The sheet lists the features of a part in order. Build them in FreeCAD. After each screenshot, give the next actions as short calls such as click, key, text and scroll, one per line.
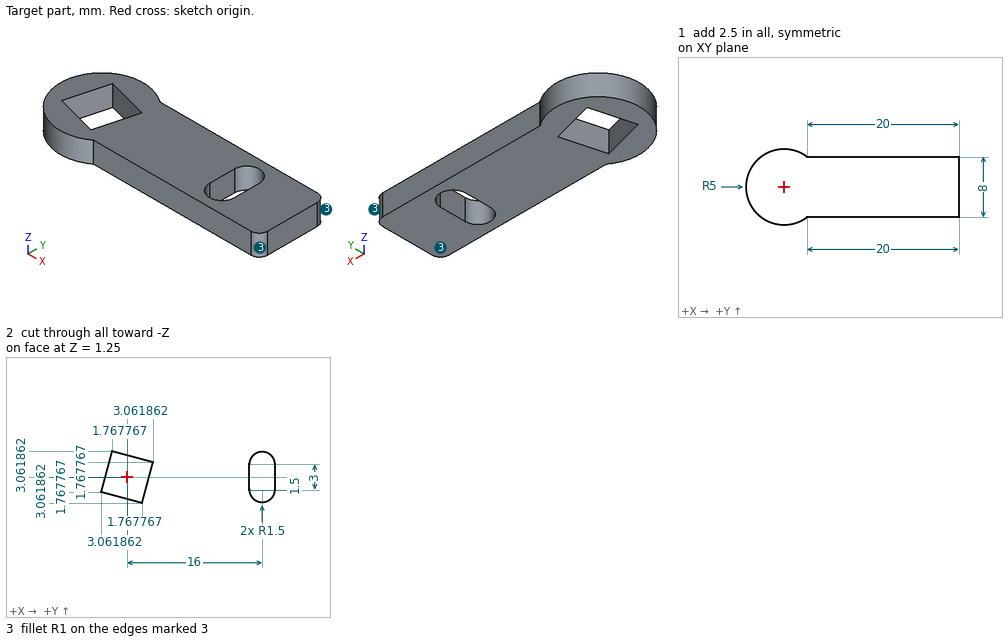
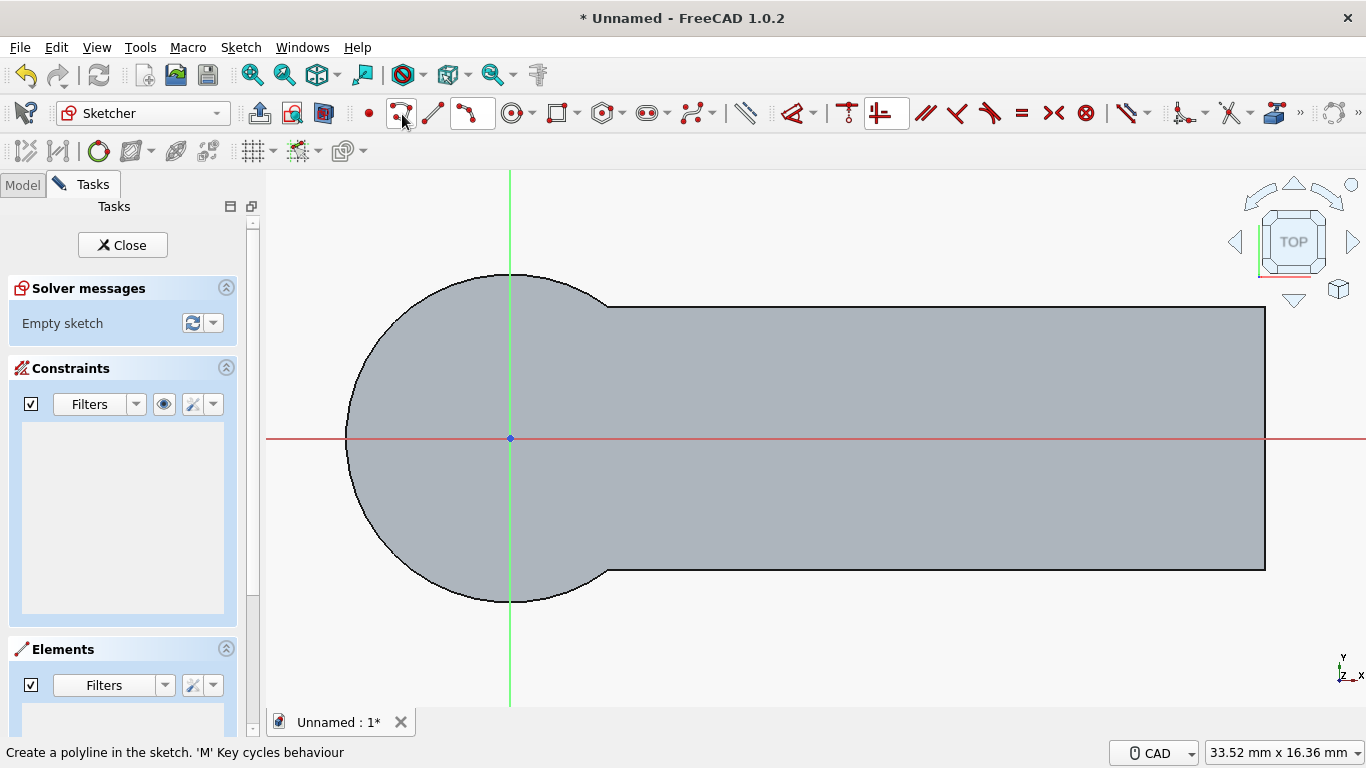
click(568, 539)
click(611, 380)
click(452, 338)
click(410, 497)
click(568, 540)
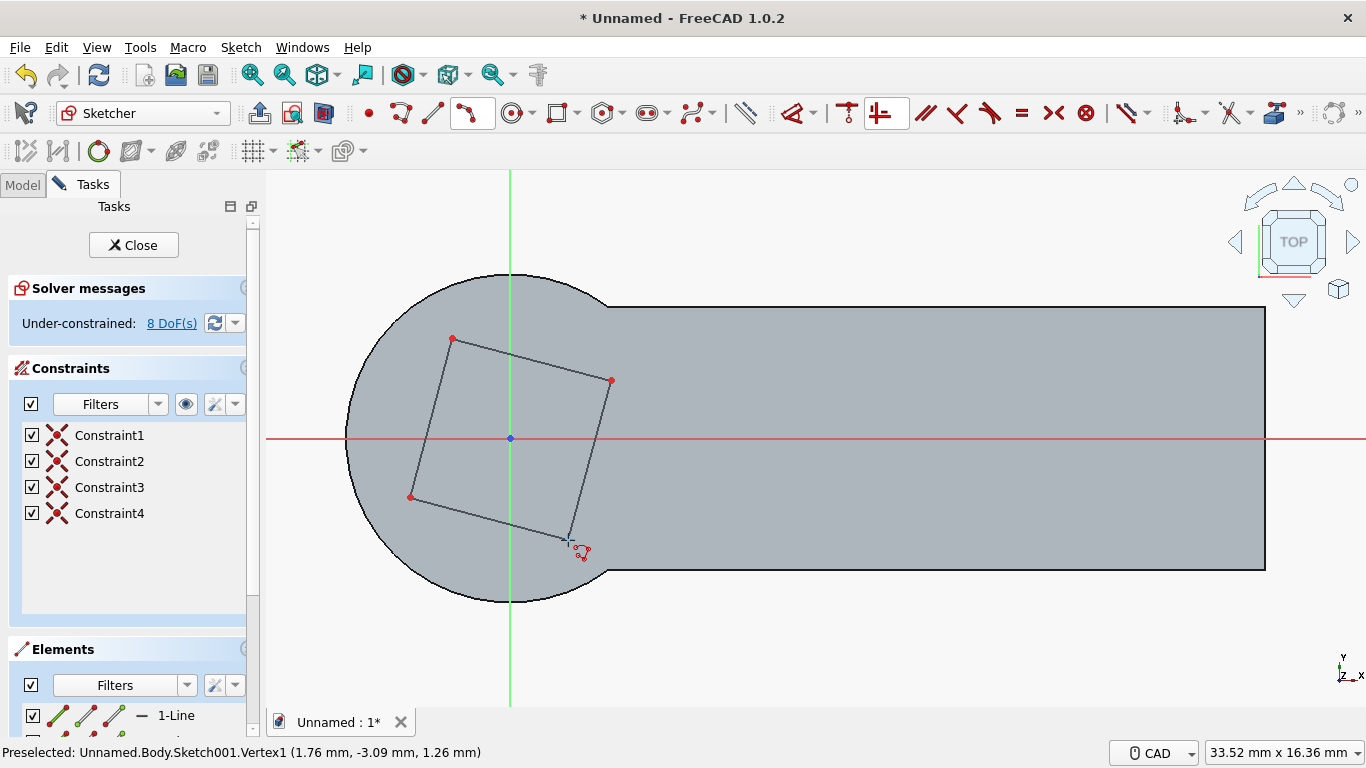
click(648, 114)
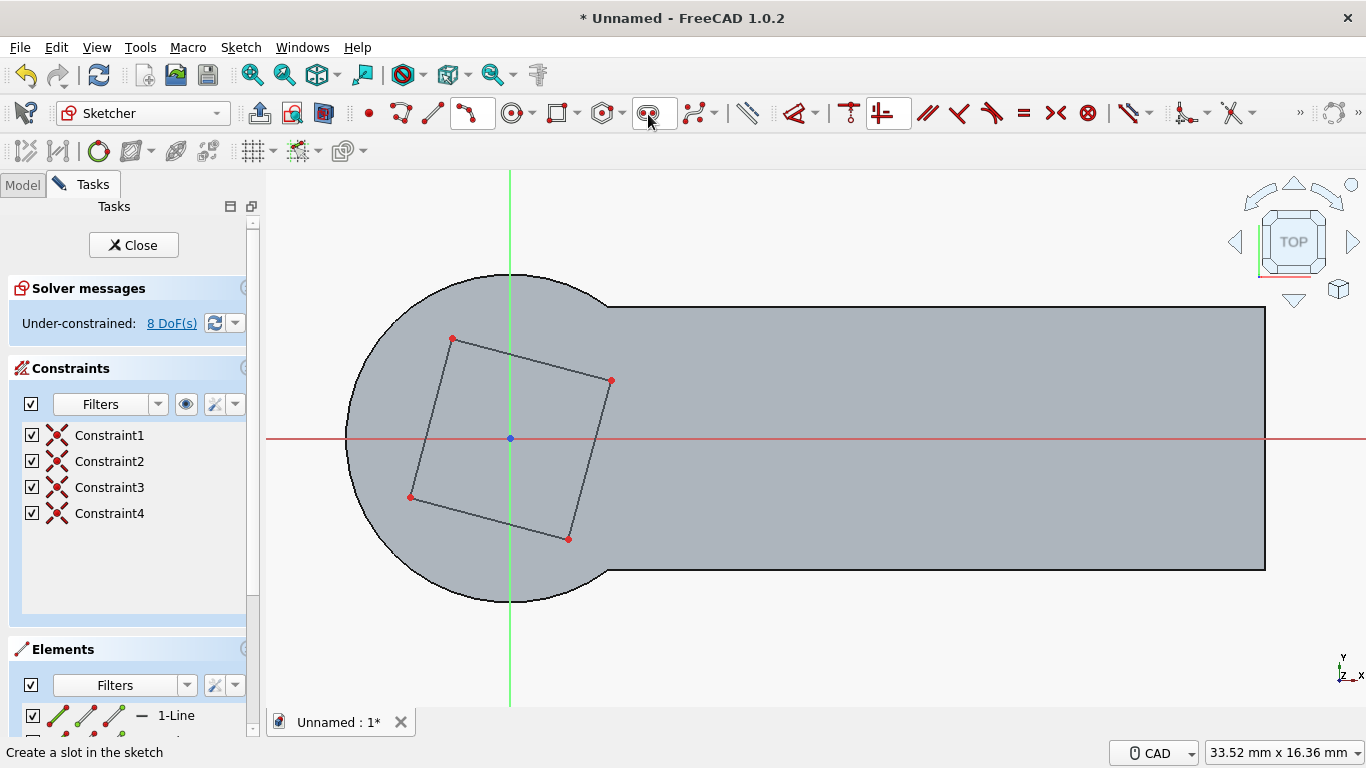
click(1035, 488)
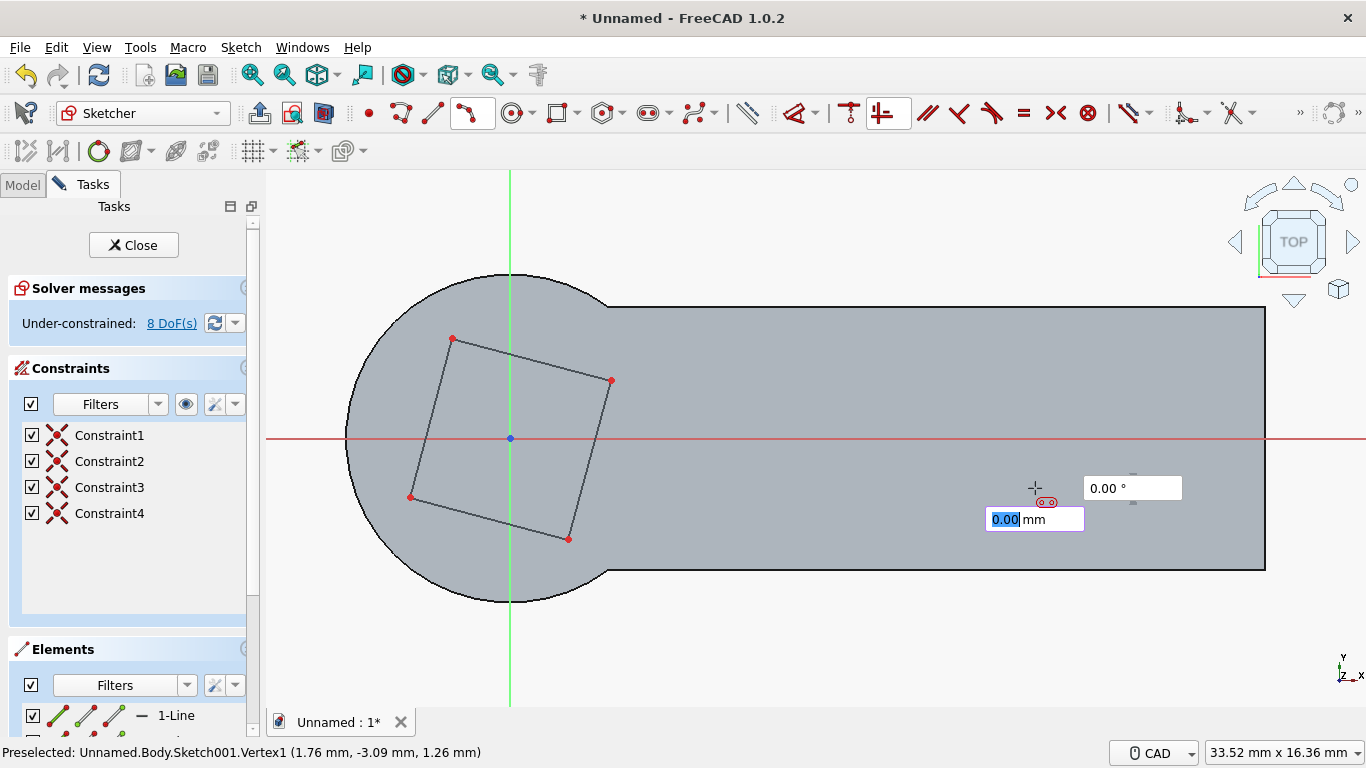
click(1035, 389)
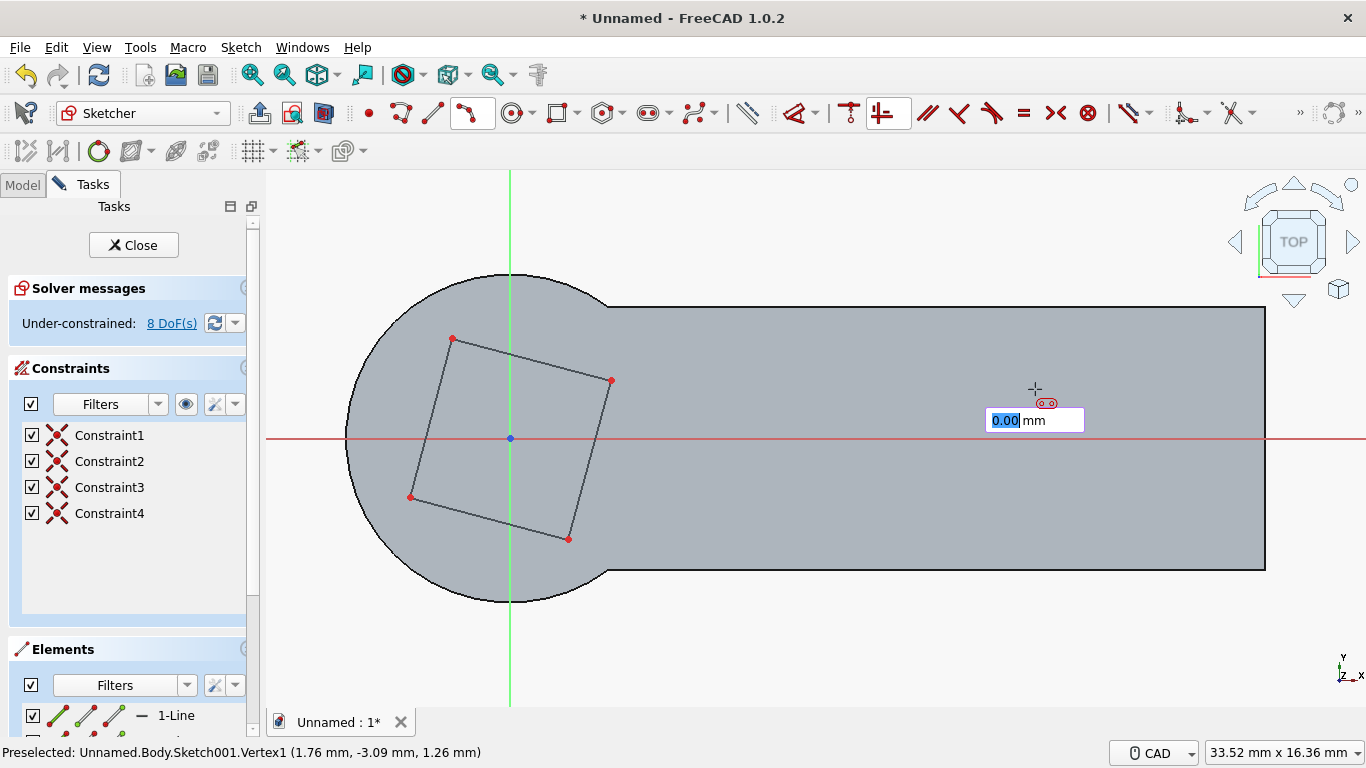
click(986, 424)
key(Escape)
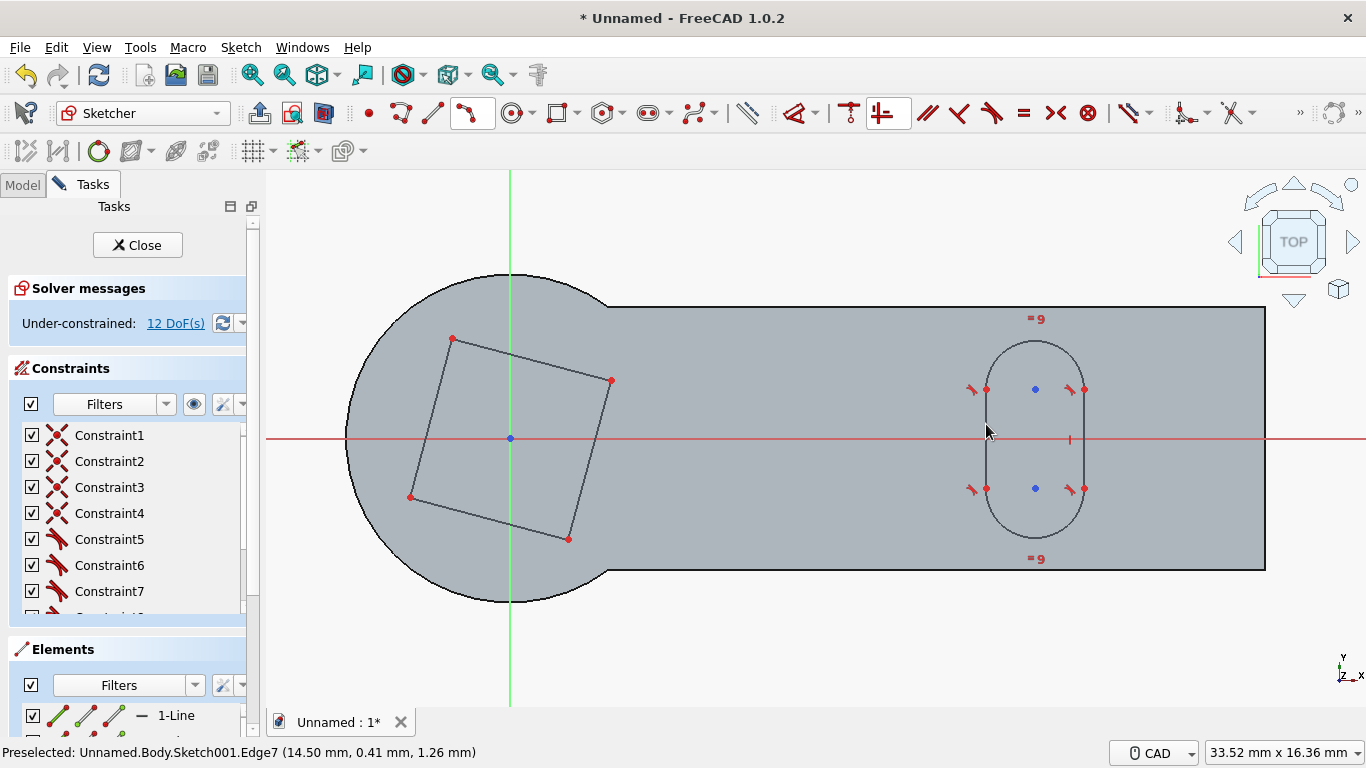
click(794, 114)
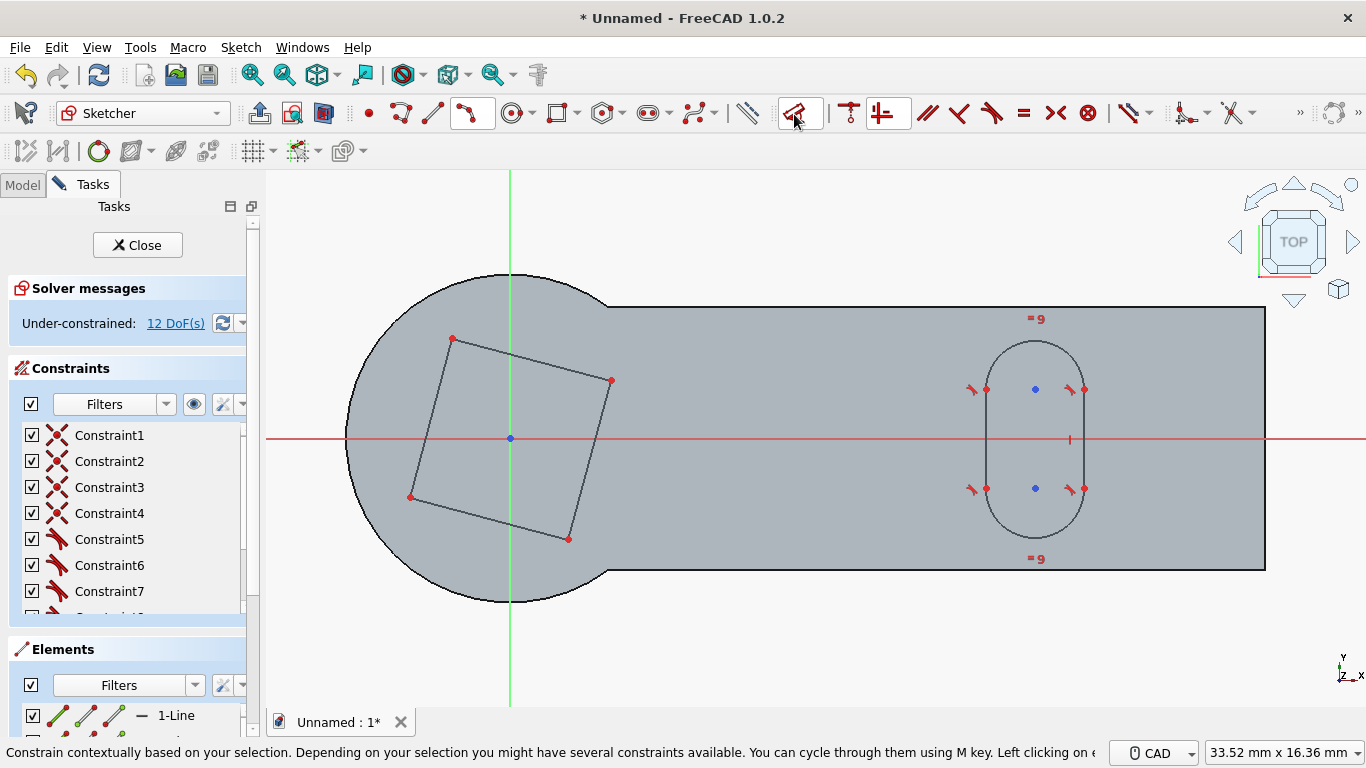
click(1006, 529)
click(987, 555)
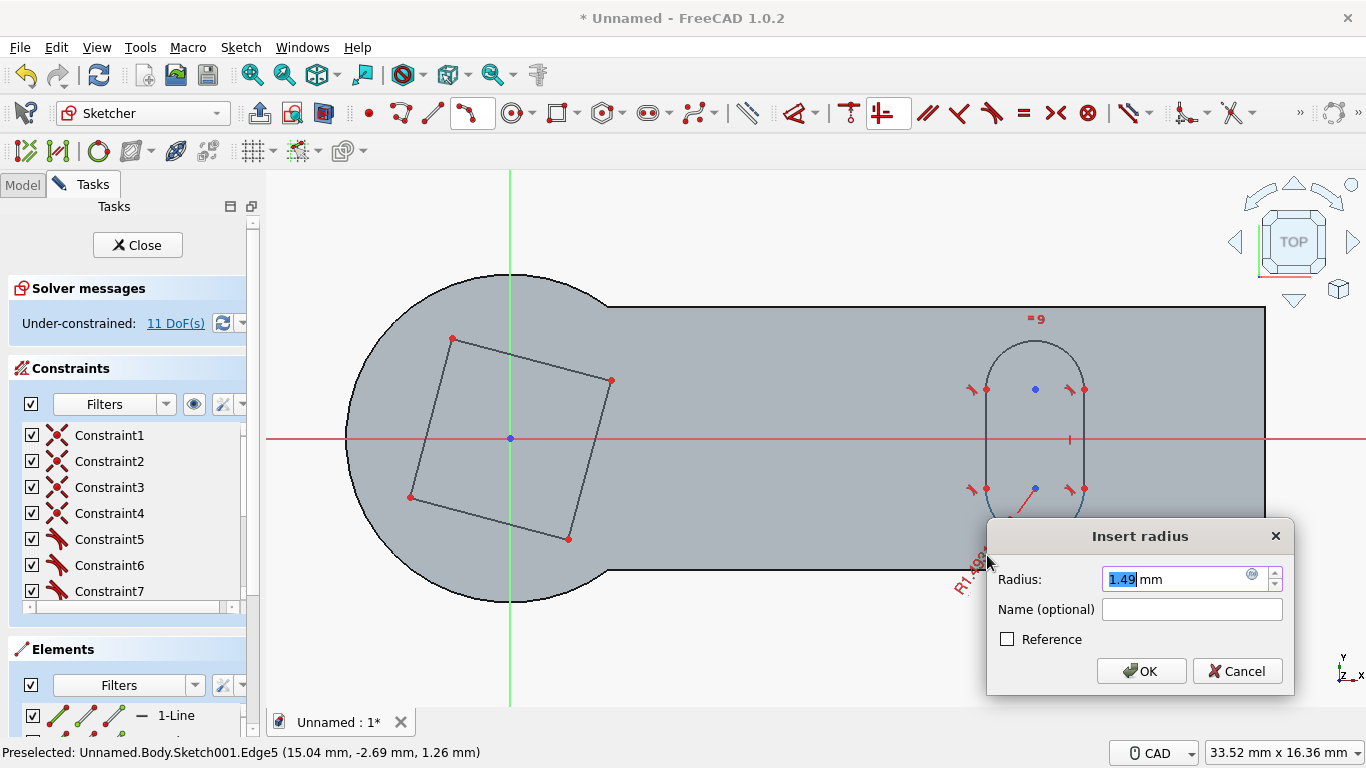
text(1.5)
key(Return)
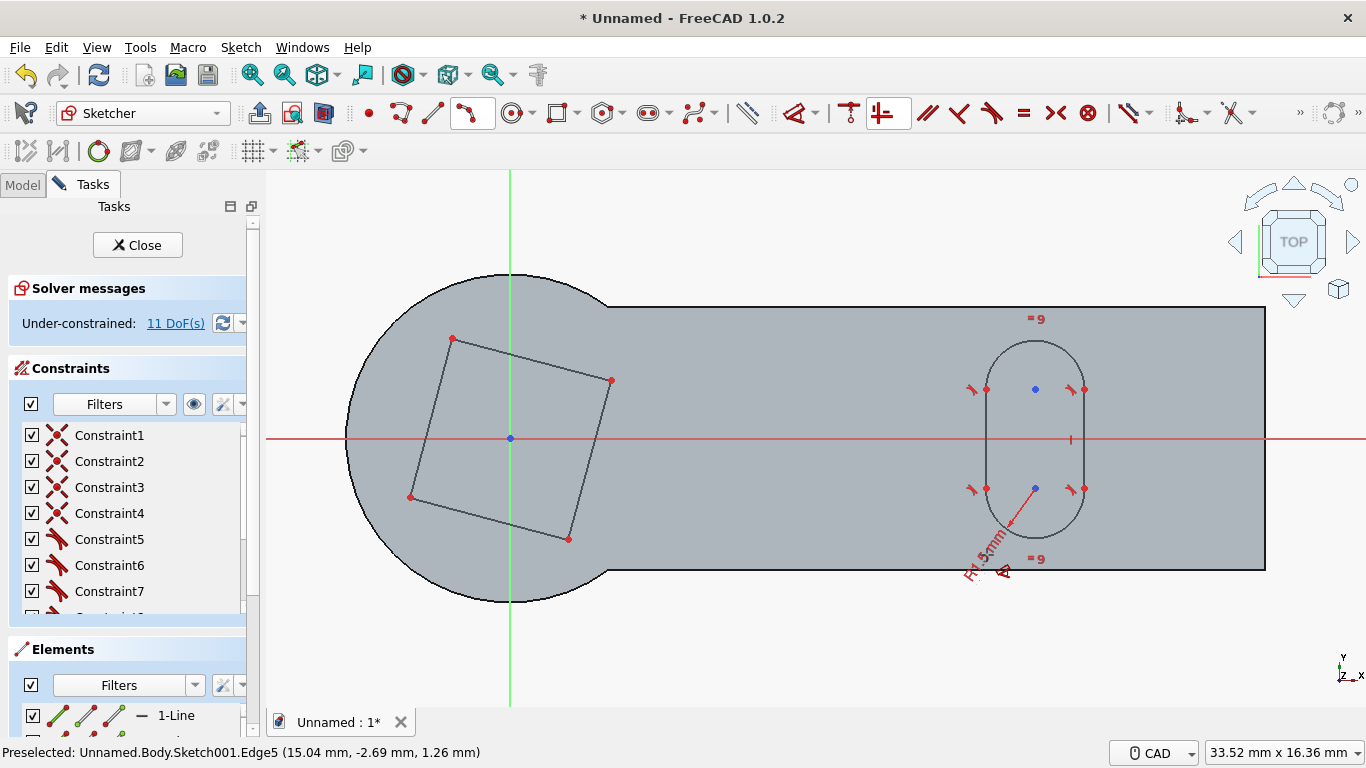
click(986, 459)
click(1020, 417)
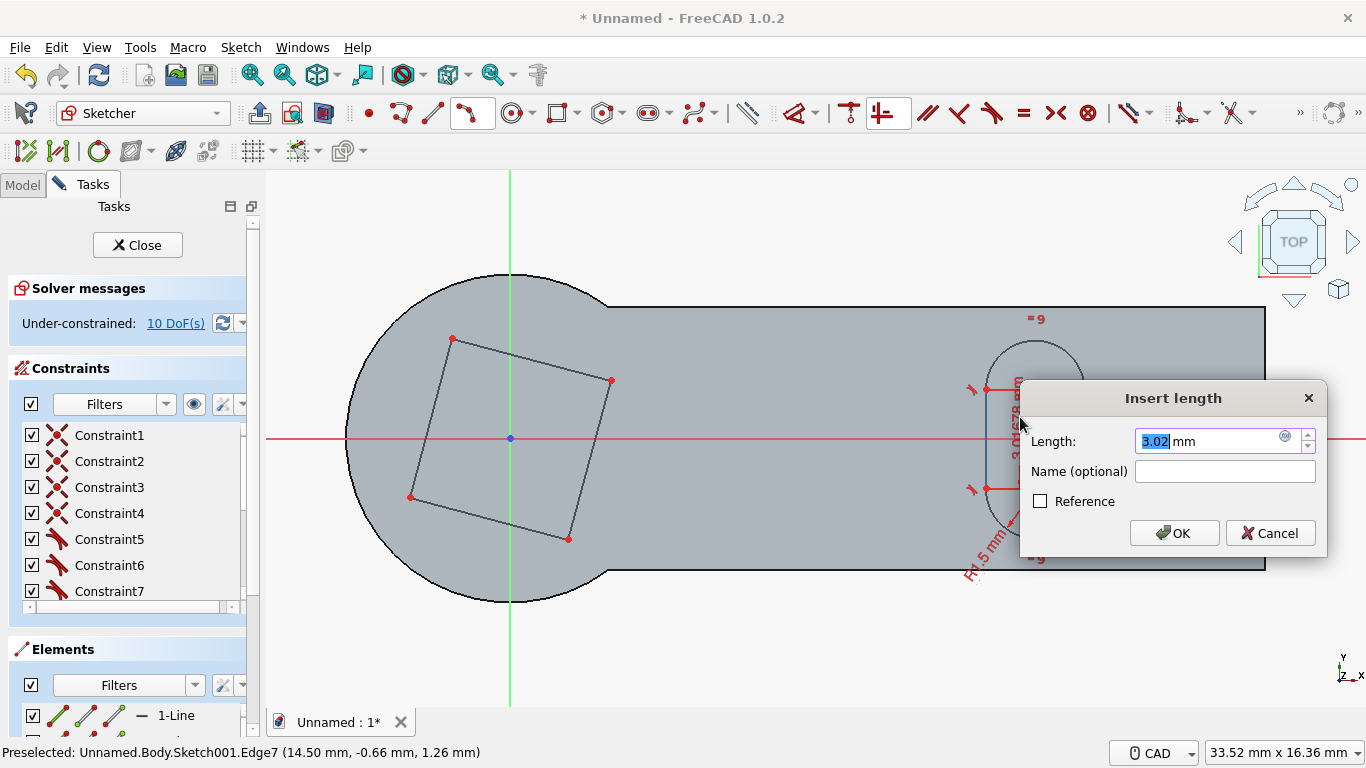
text(3)
key(Return)